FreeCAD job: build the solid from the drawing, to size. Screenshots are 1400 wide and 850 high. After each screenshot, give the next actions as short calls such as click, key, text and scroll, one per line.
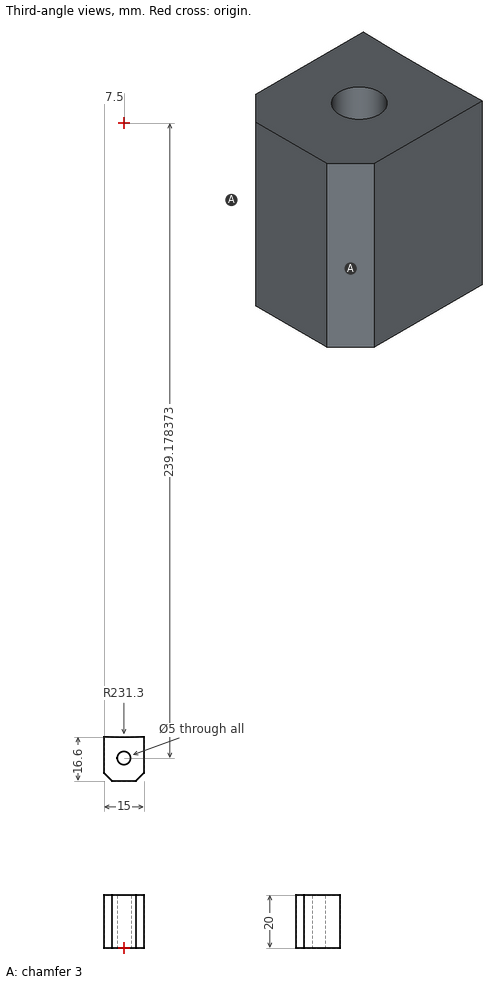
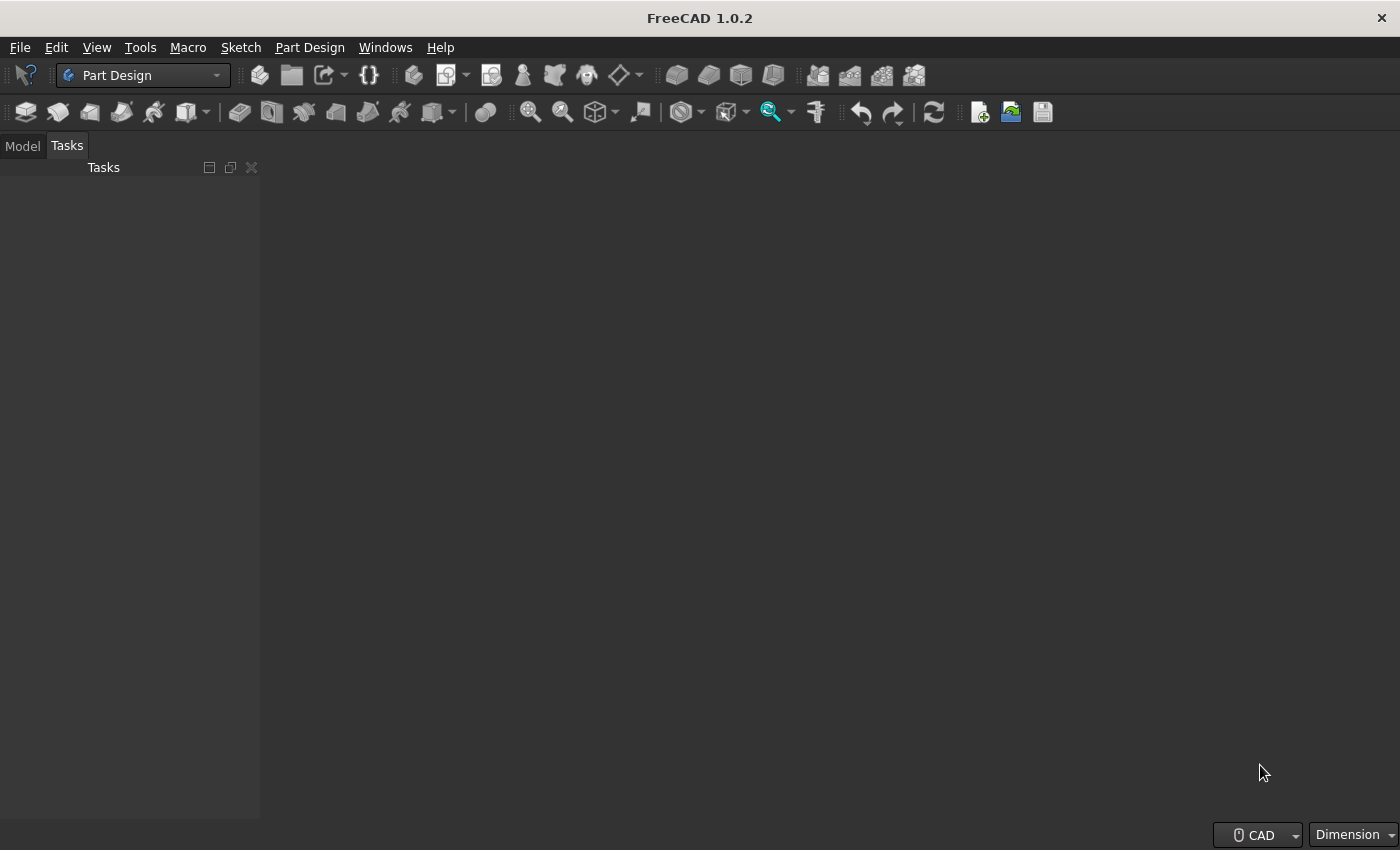
click(980, 112)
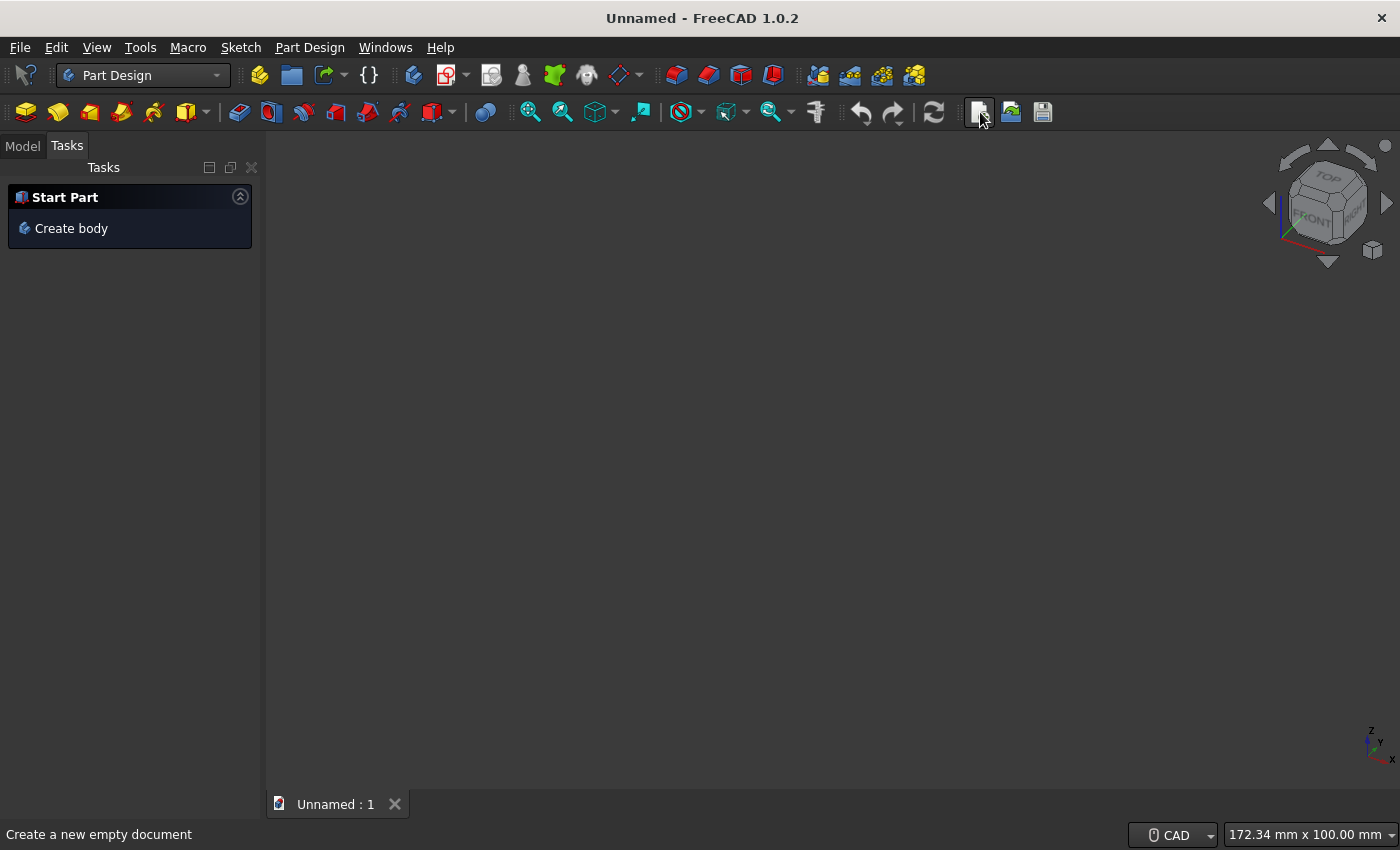
click(446, 76)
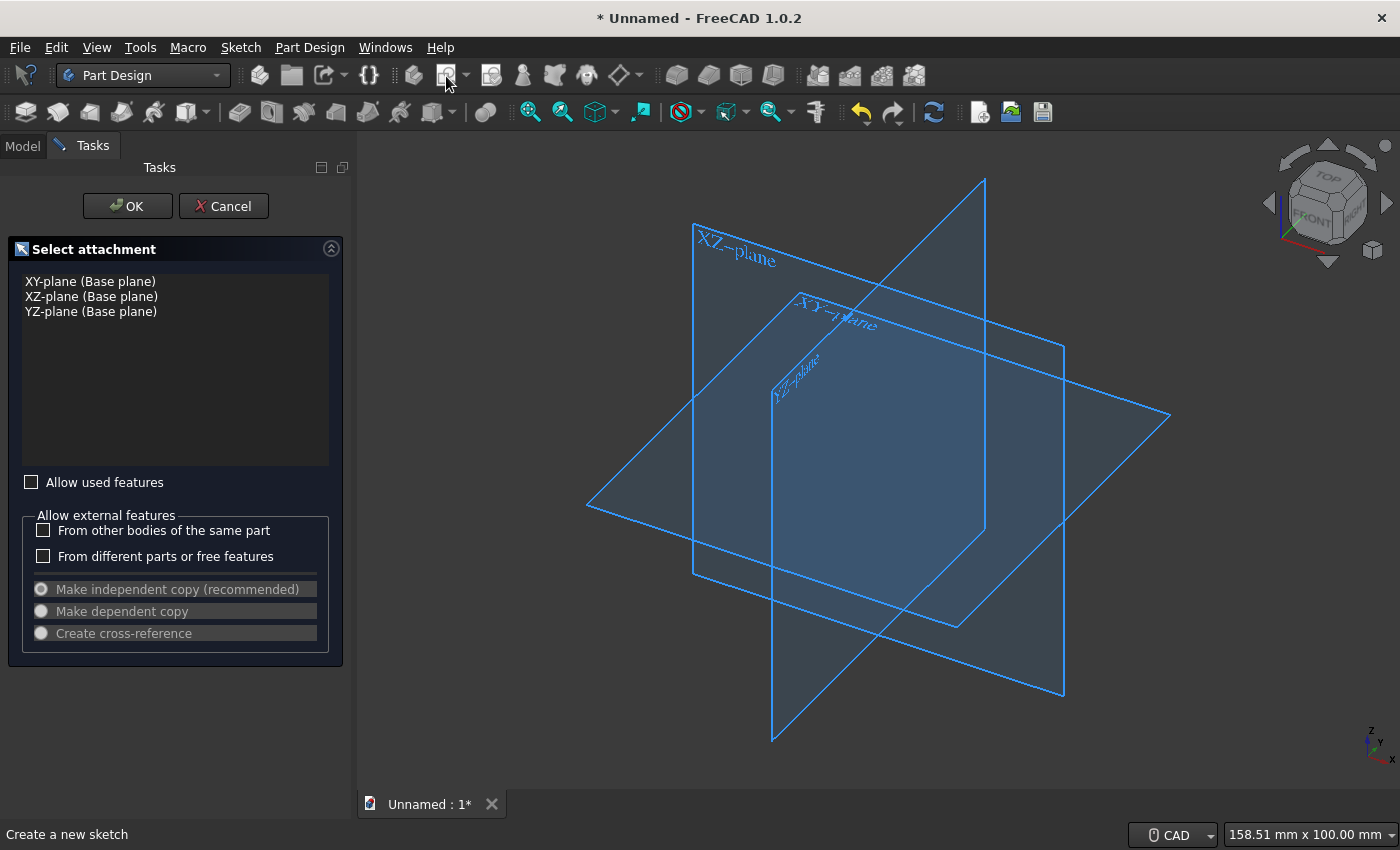
click(82, 282)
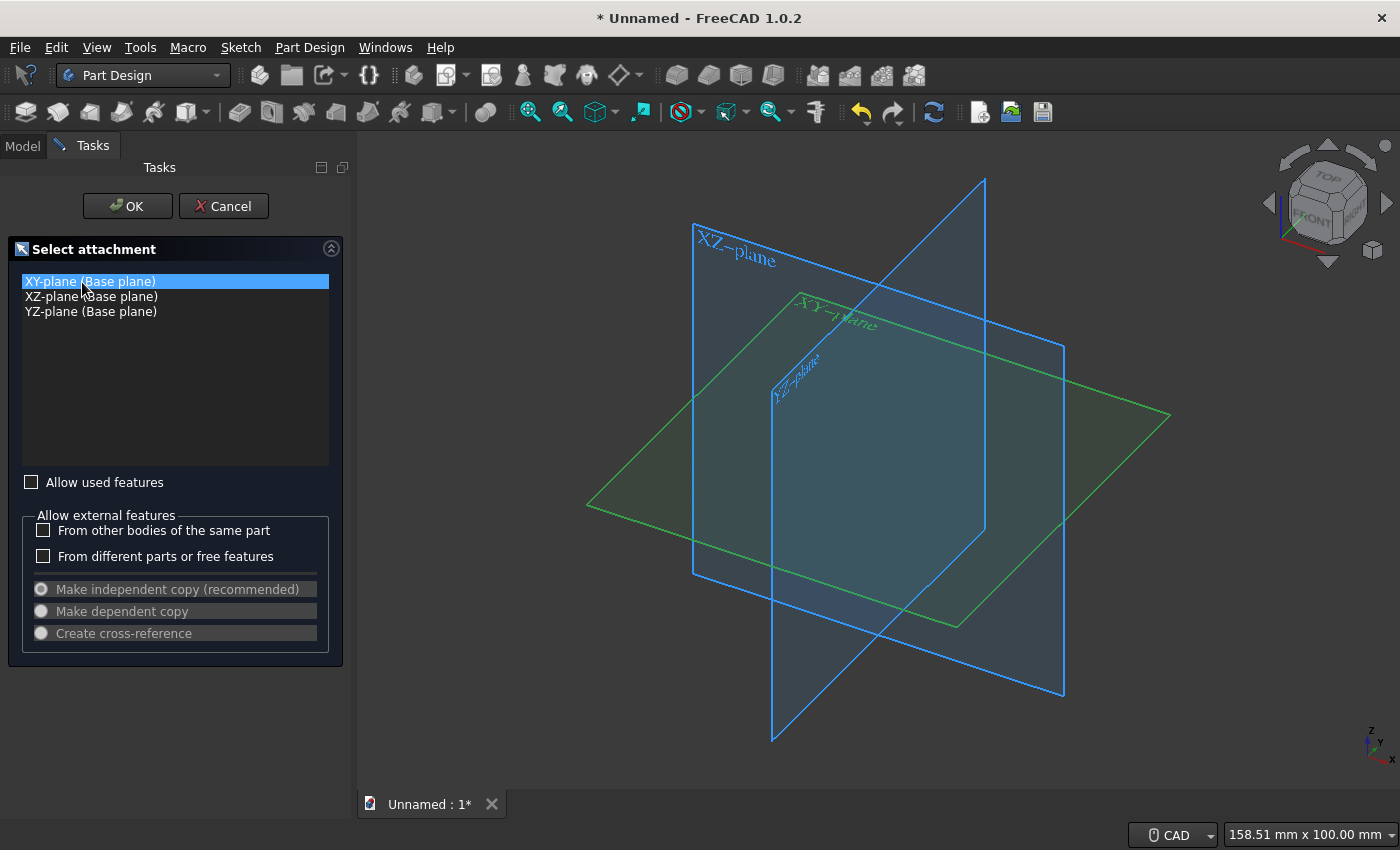
click(128, 206)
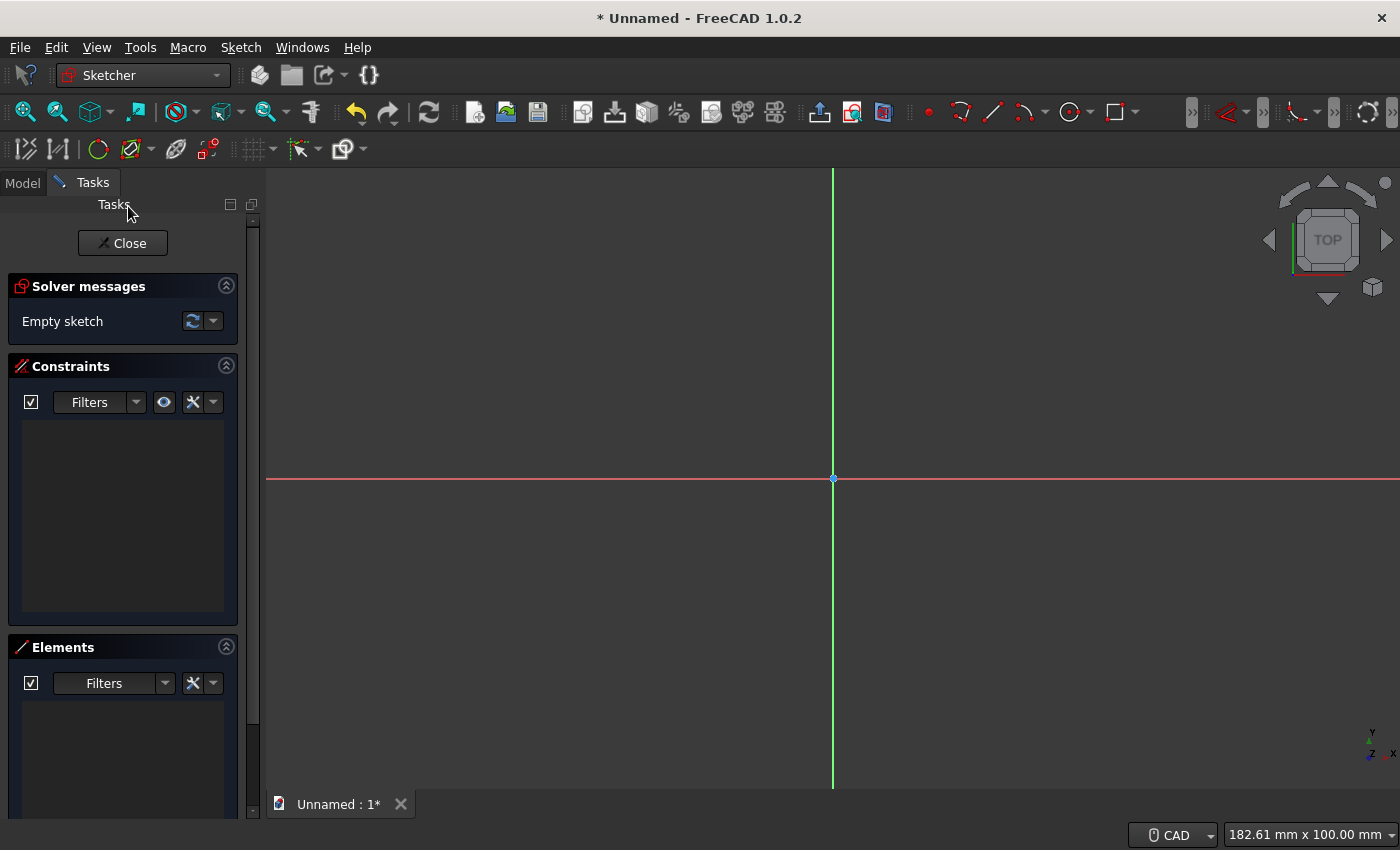
scroll(764, 478, down, 5)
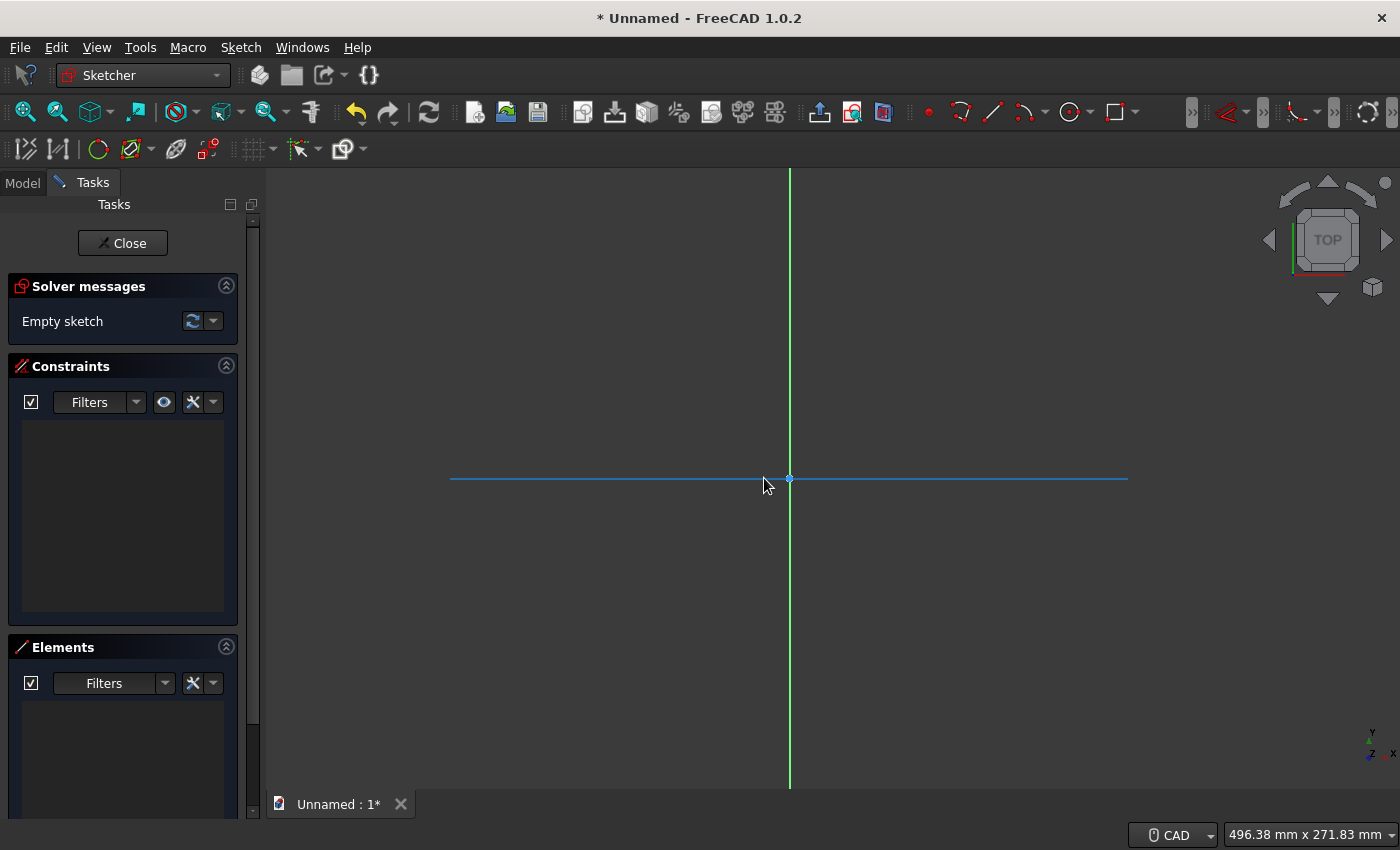
scroll(764, 478, down, 5)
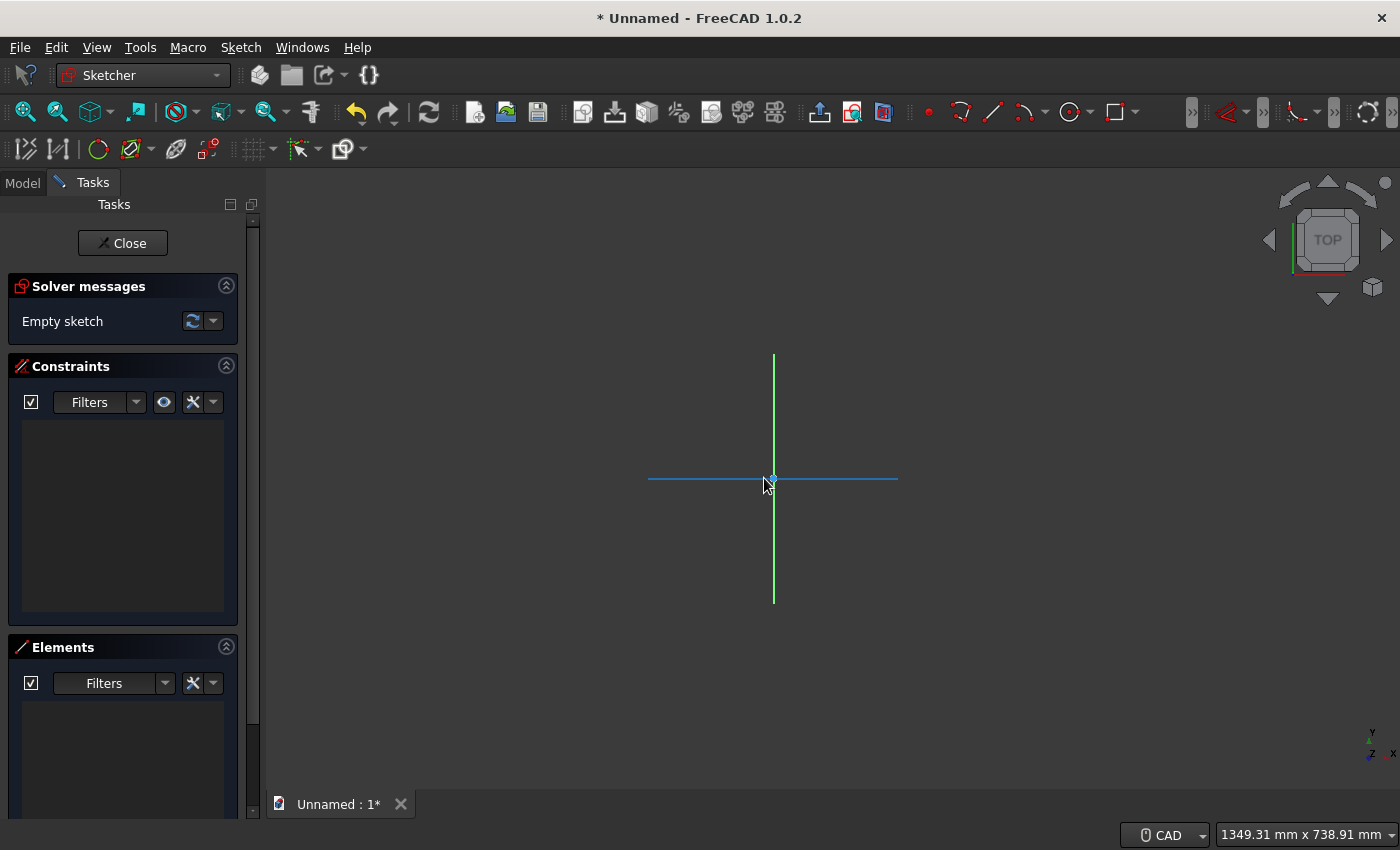
scroll(774, 690, up, 15)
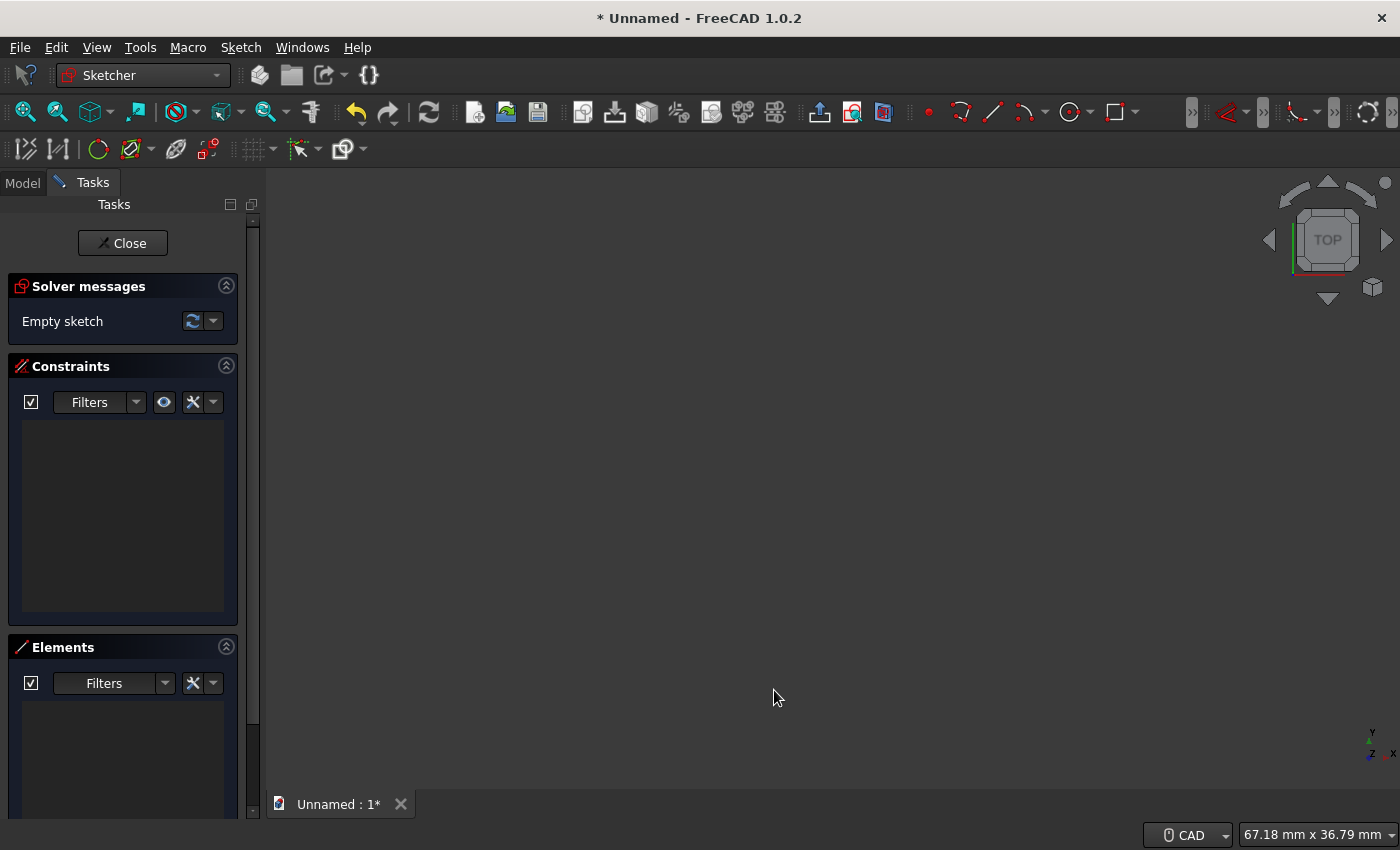
scroll(750, 448, up, 2)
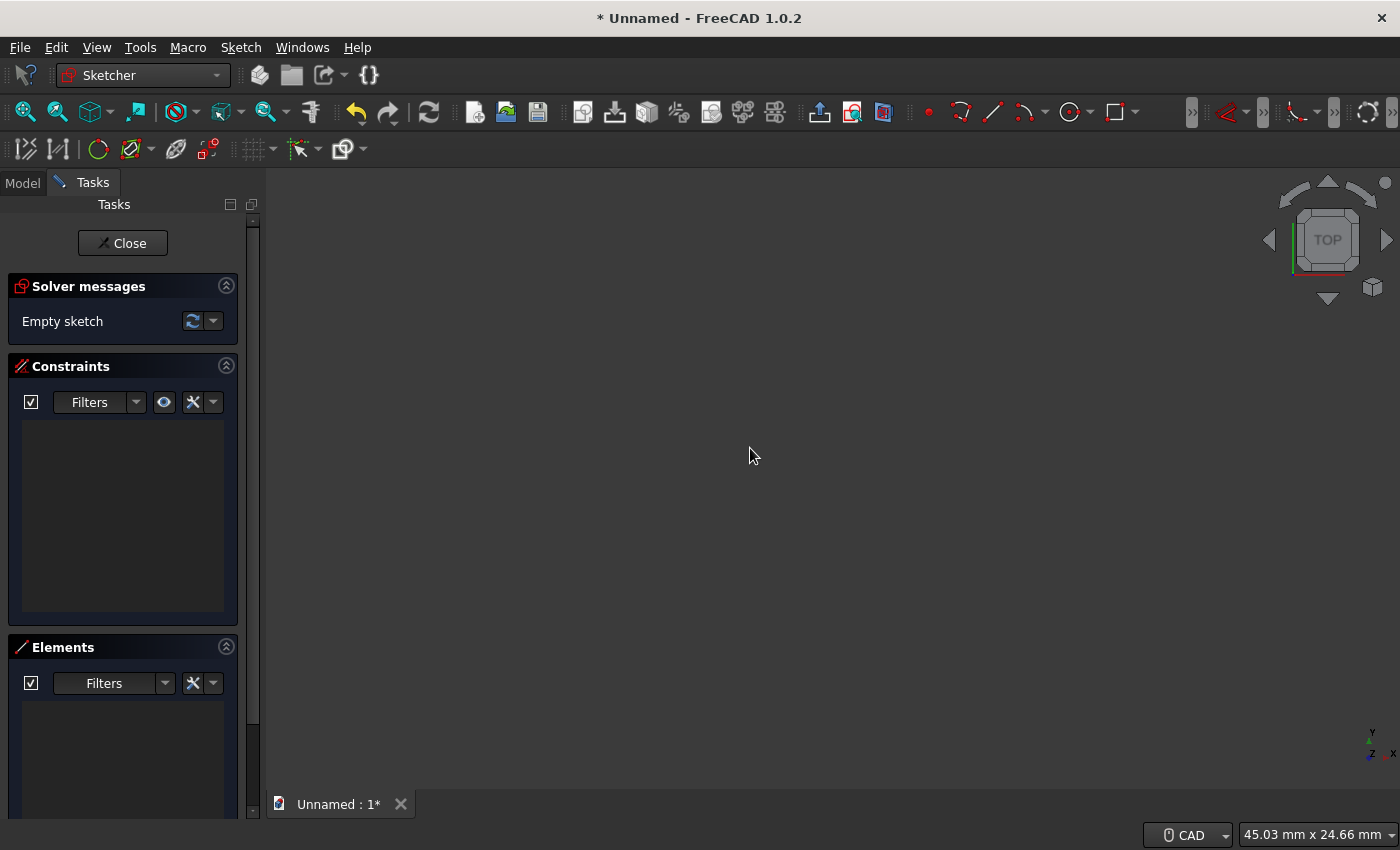
click(962, 112)